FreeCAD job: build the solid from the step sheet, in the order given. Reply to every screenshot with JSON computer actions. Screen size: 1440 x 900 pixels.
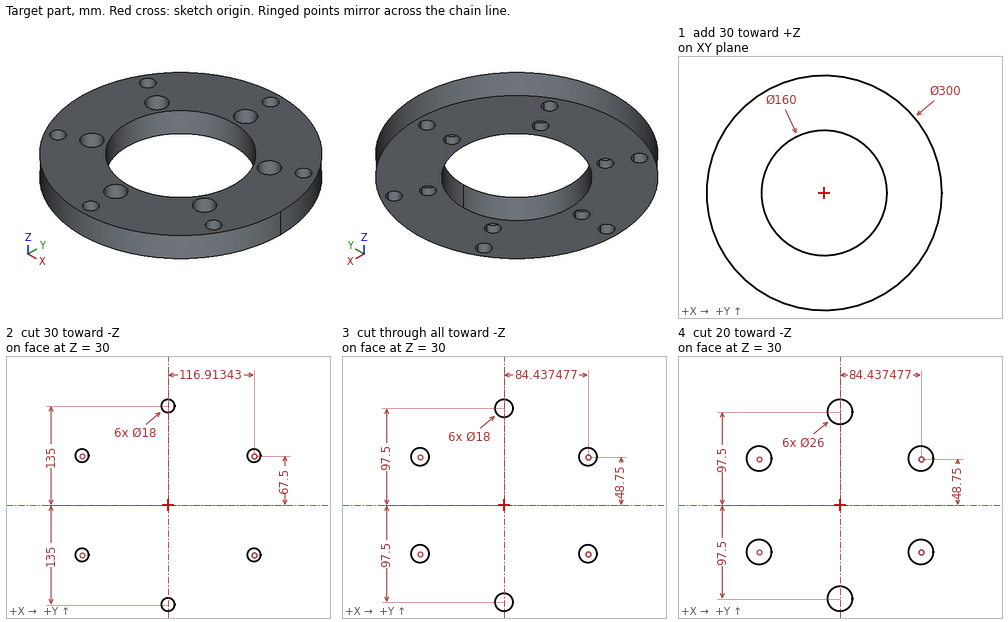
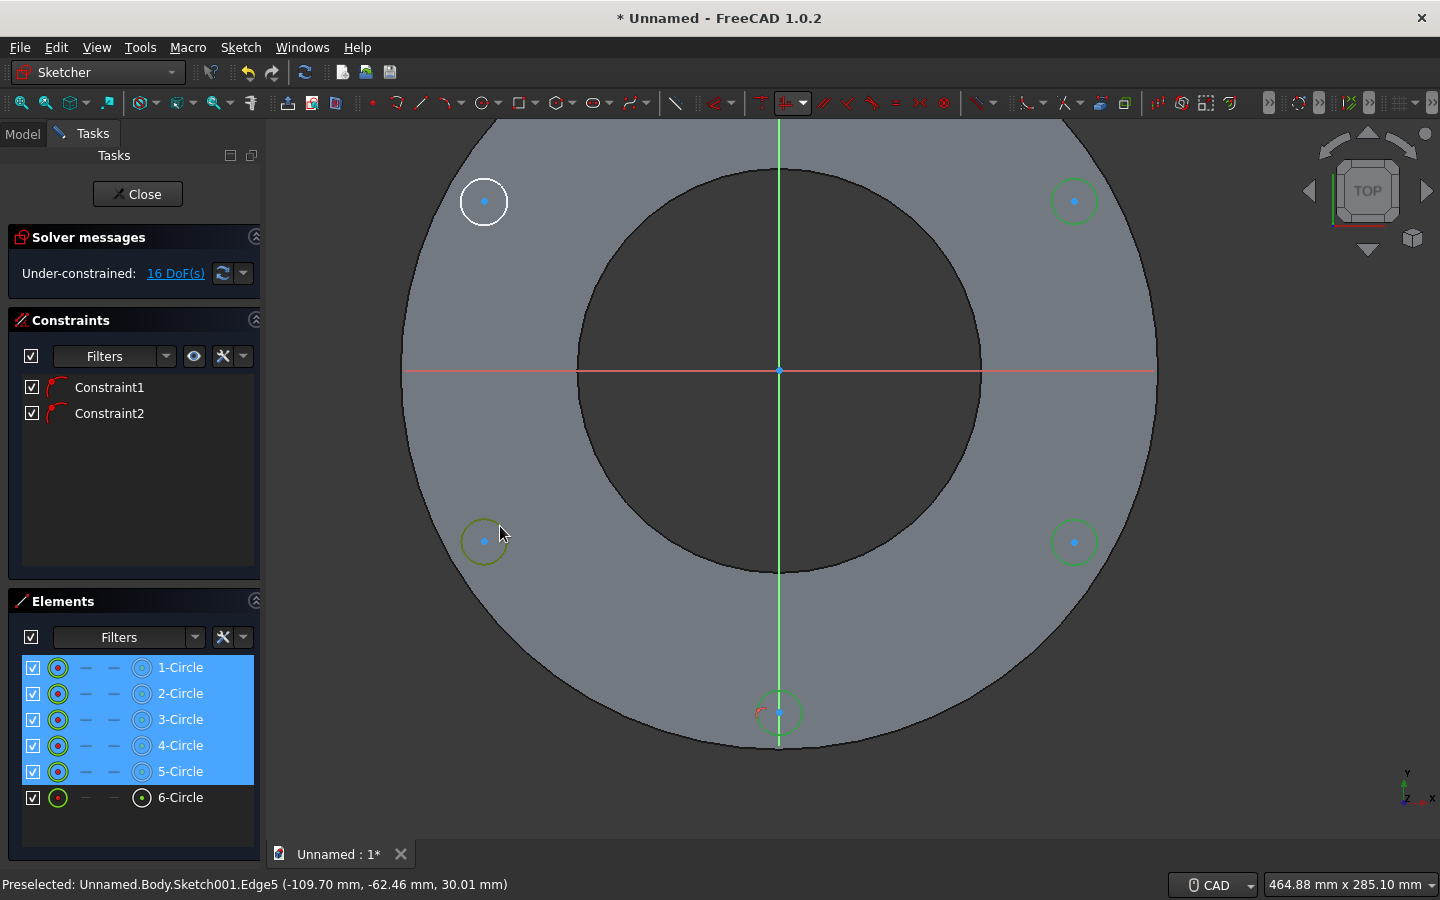
{"action": "left_click", "coordinate": [501, 185]}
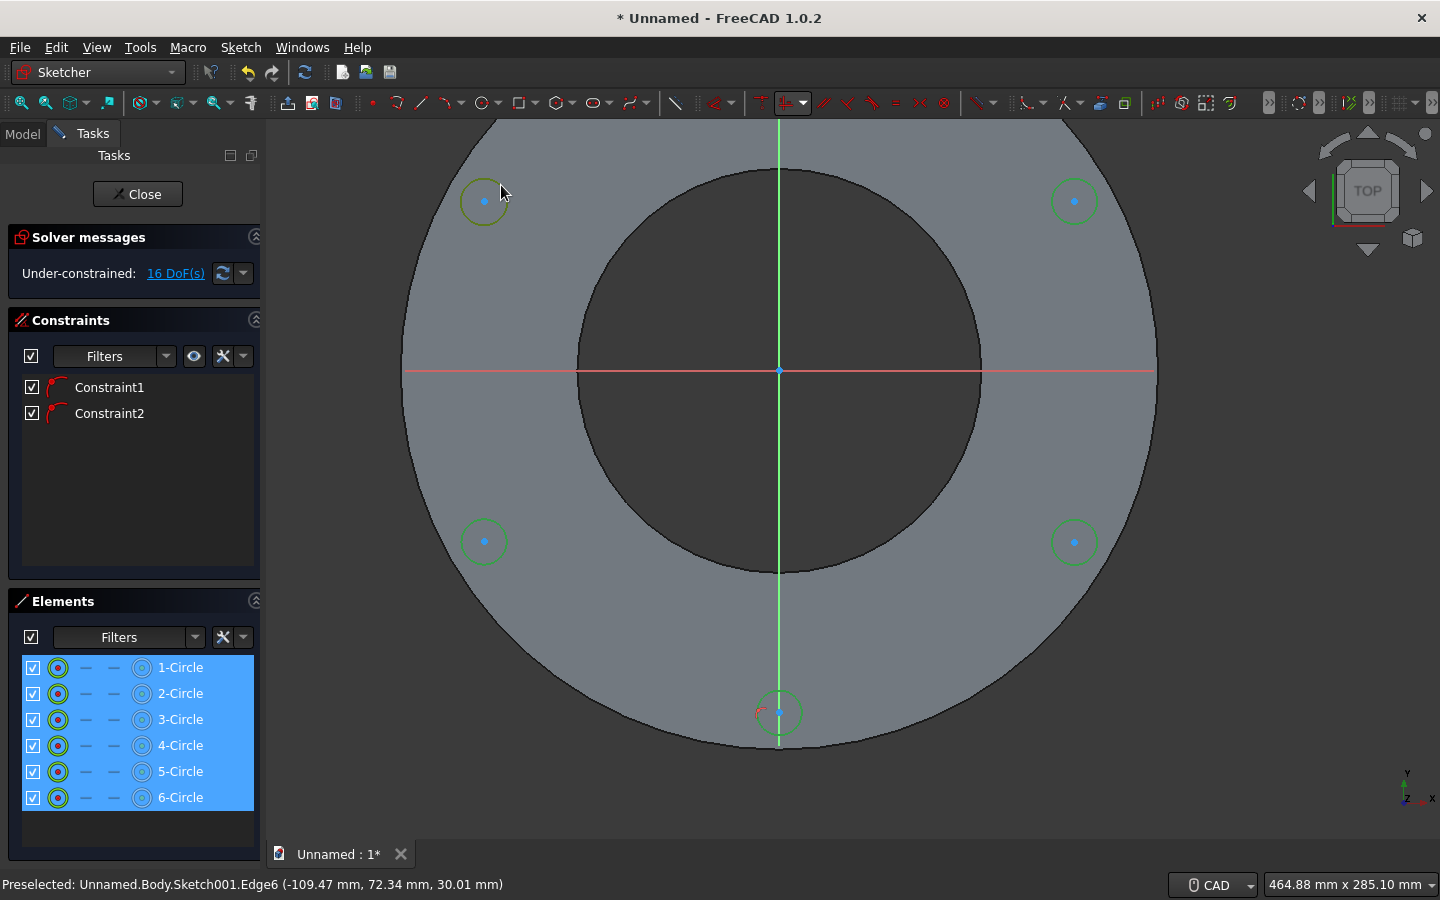
{"action": "left_click", "coordinate": [896, 104]}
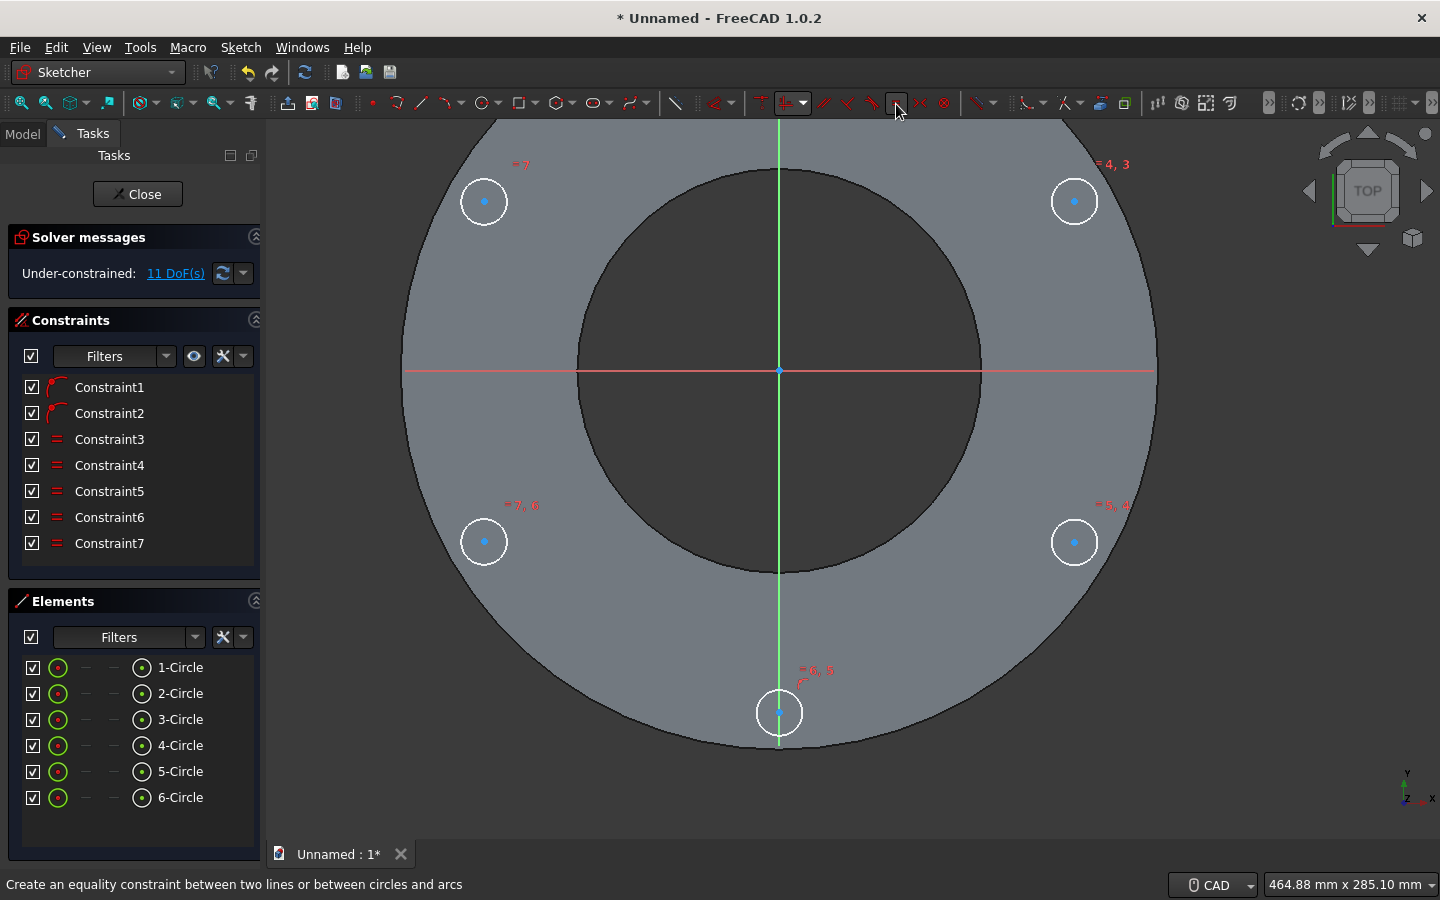
{"action": "left_click", "coordinate": [1075, 201]}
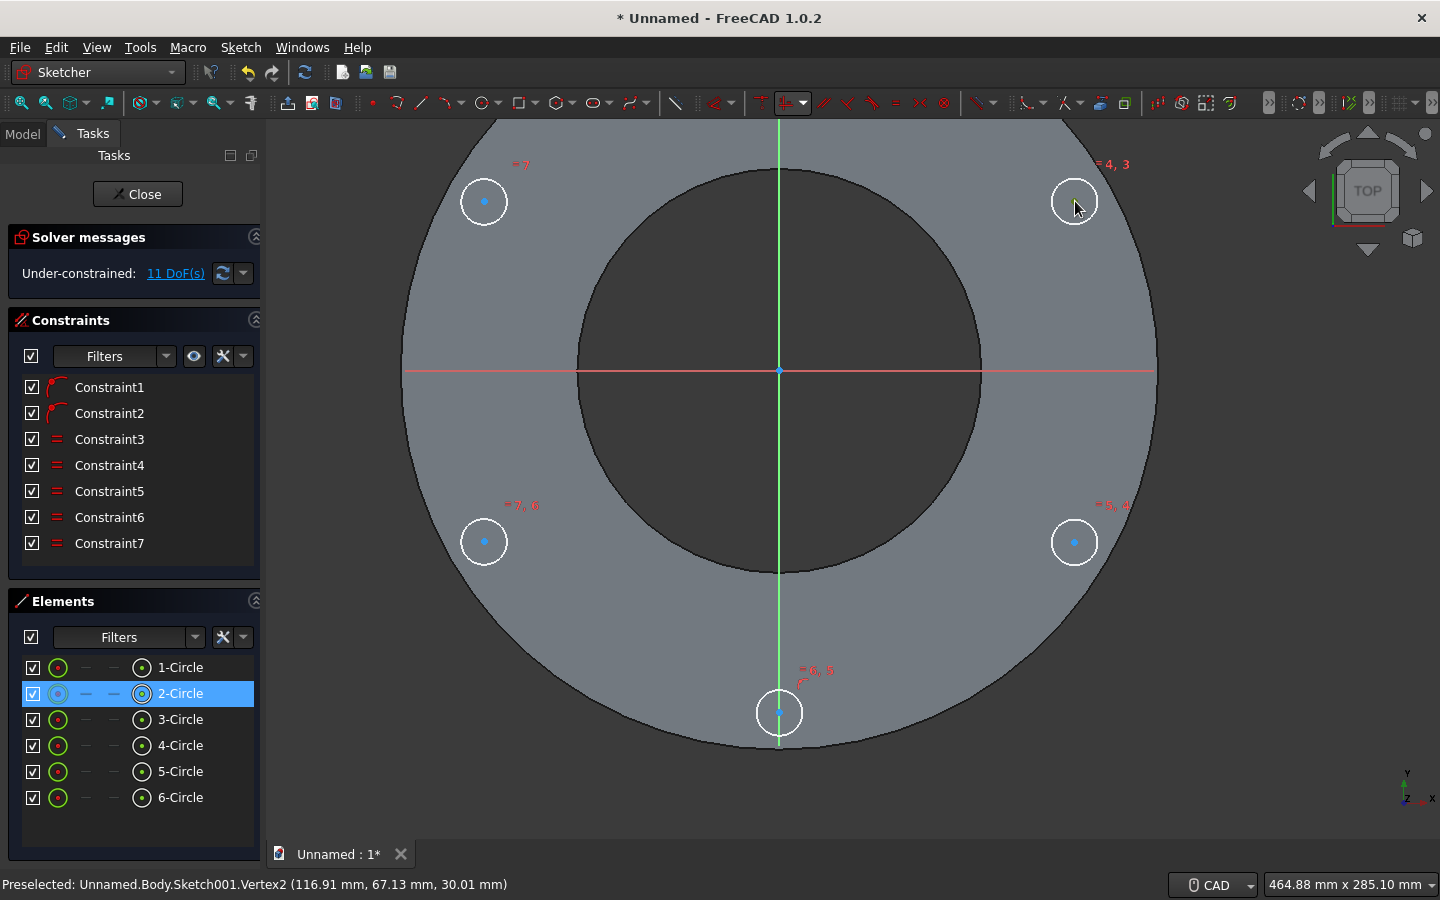
{"action": "left_click", "coordinate": [1075, 542]}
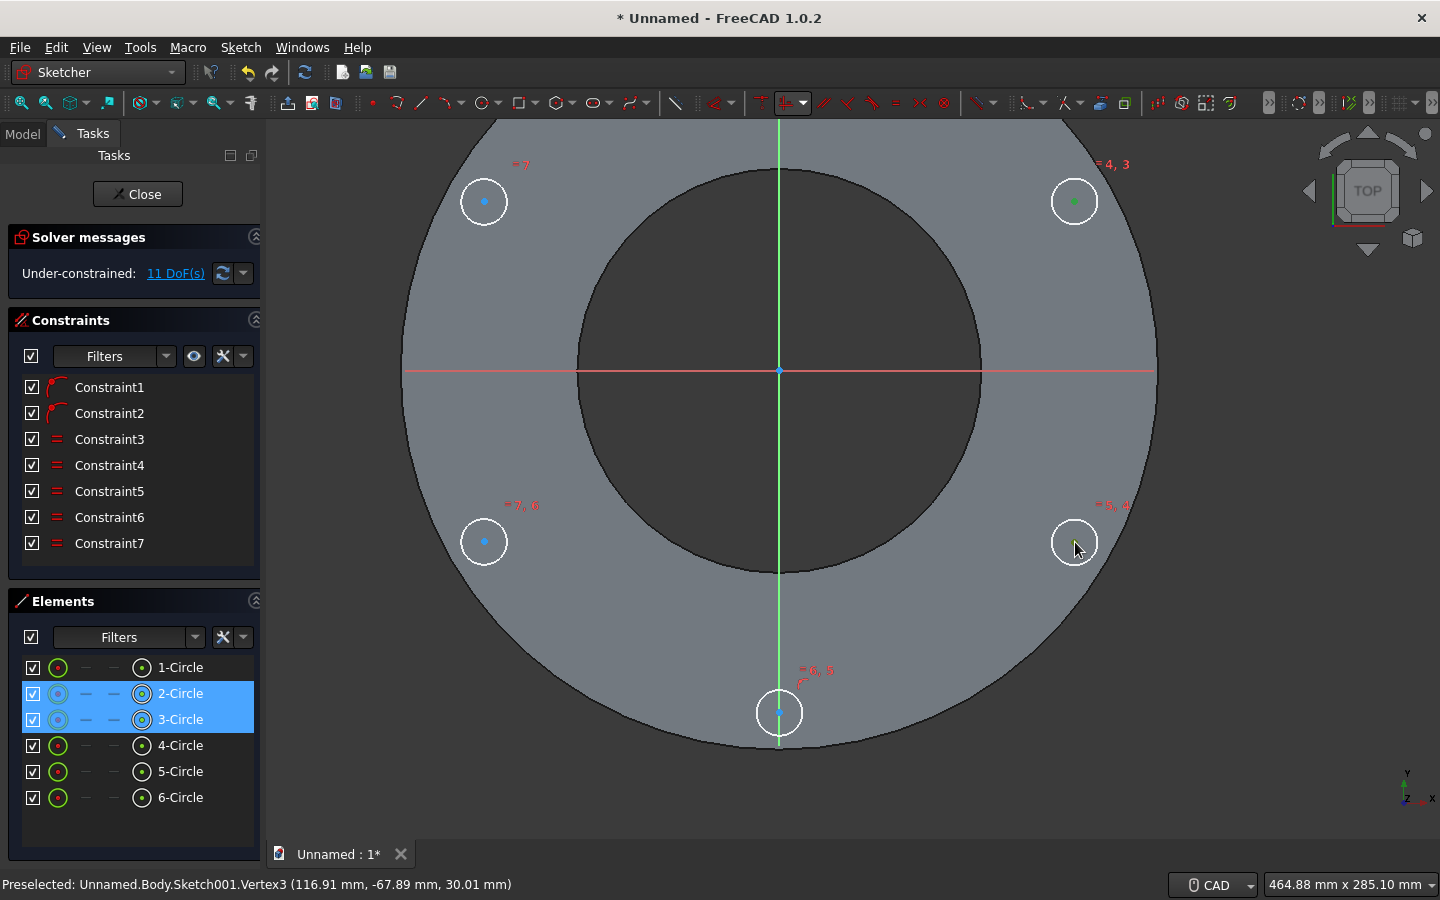
{"action": "left_click", "coordinate": [434, 371]}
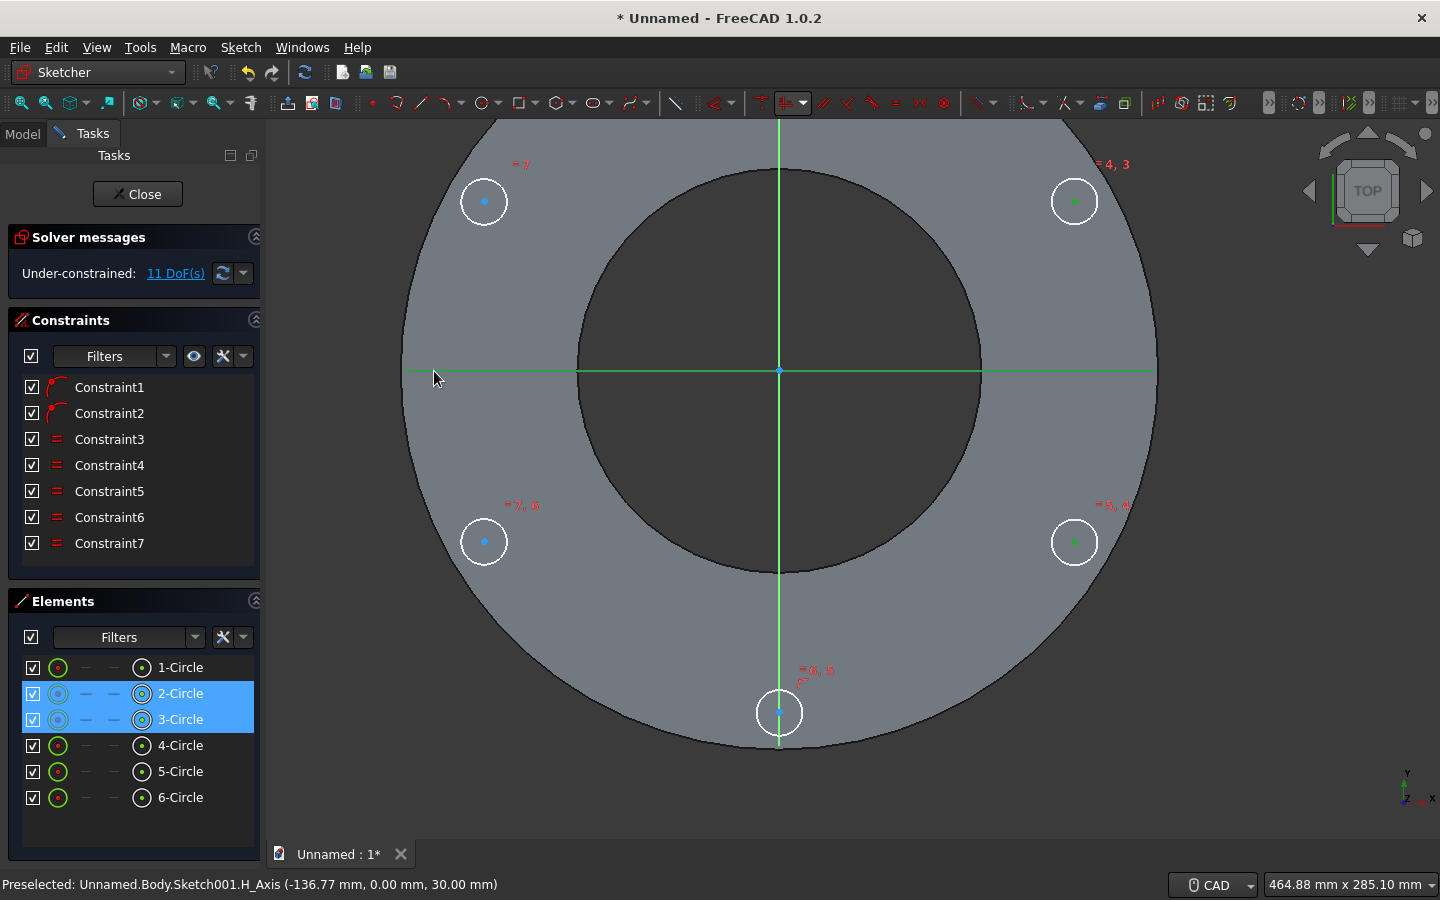
{"action": "key", "text": "s"}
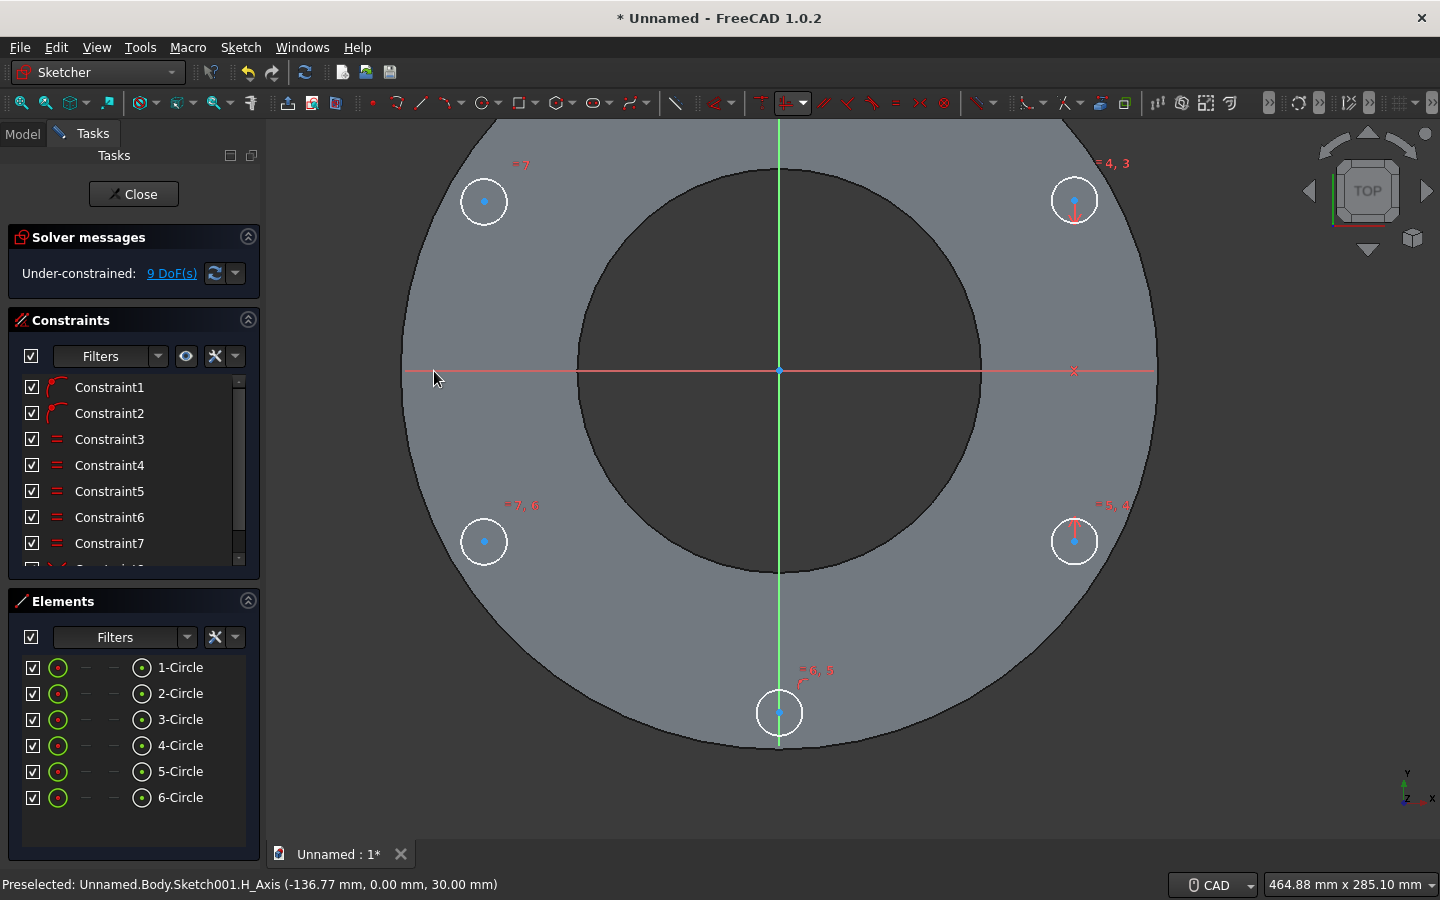
{"action": "left_click", "coordinate": [1075, 542]}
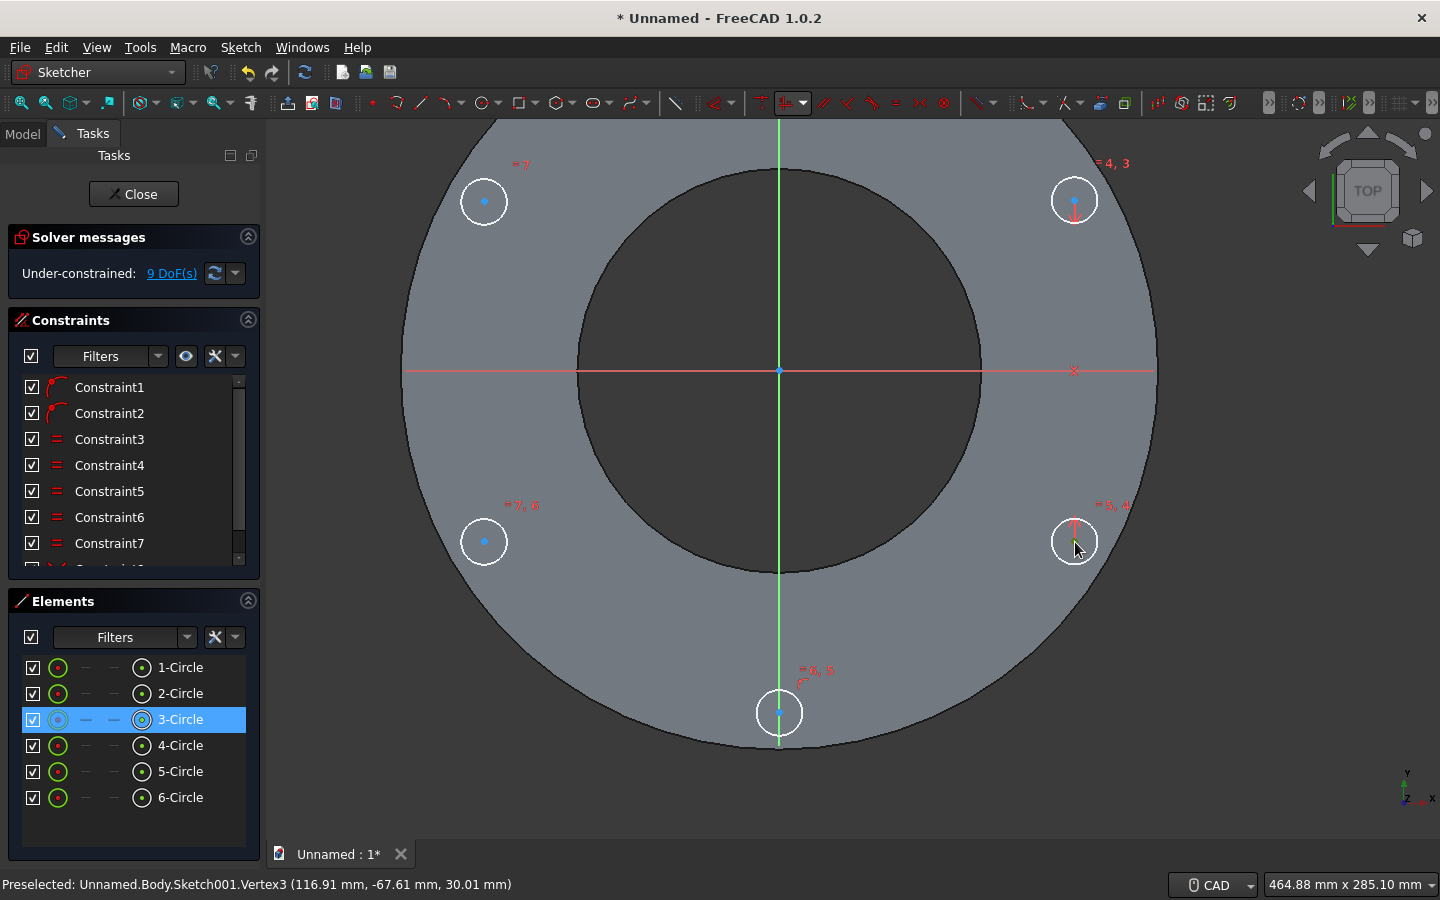
{"action": "left_click", "coordinate": [484, 542]}